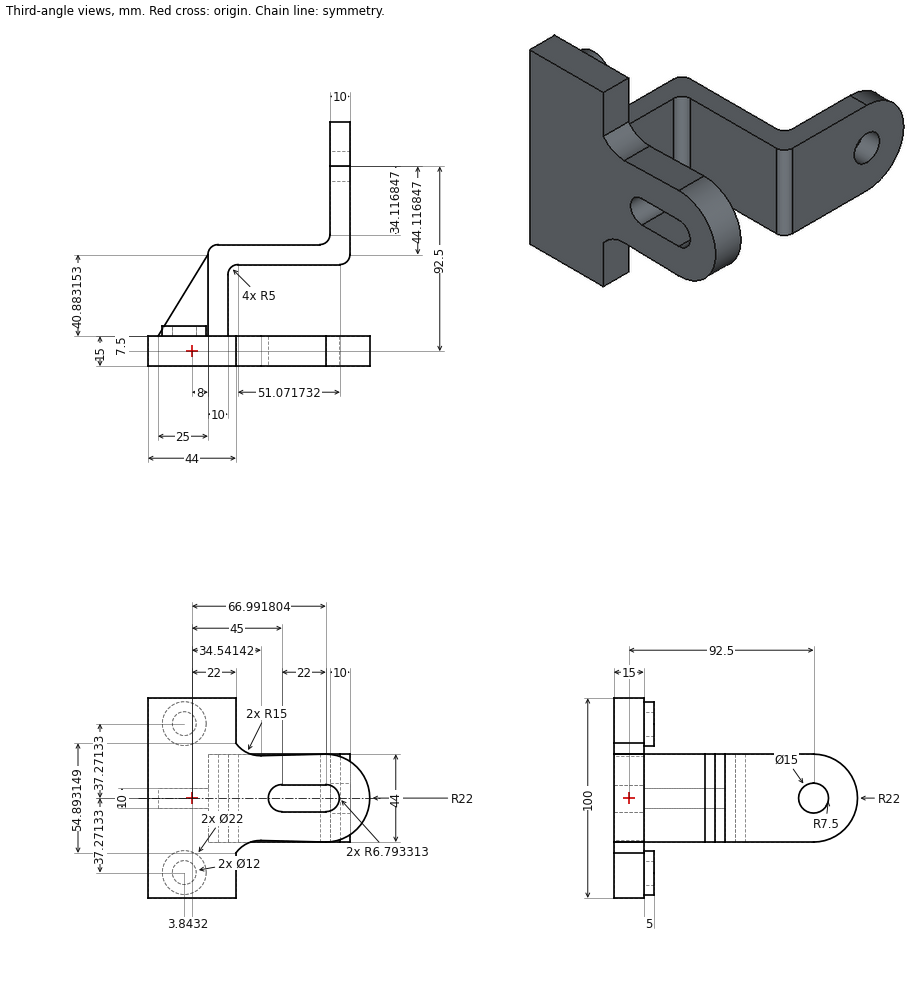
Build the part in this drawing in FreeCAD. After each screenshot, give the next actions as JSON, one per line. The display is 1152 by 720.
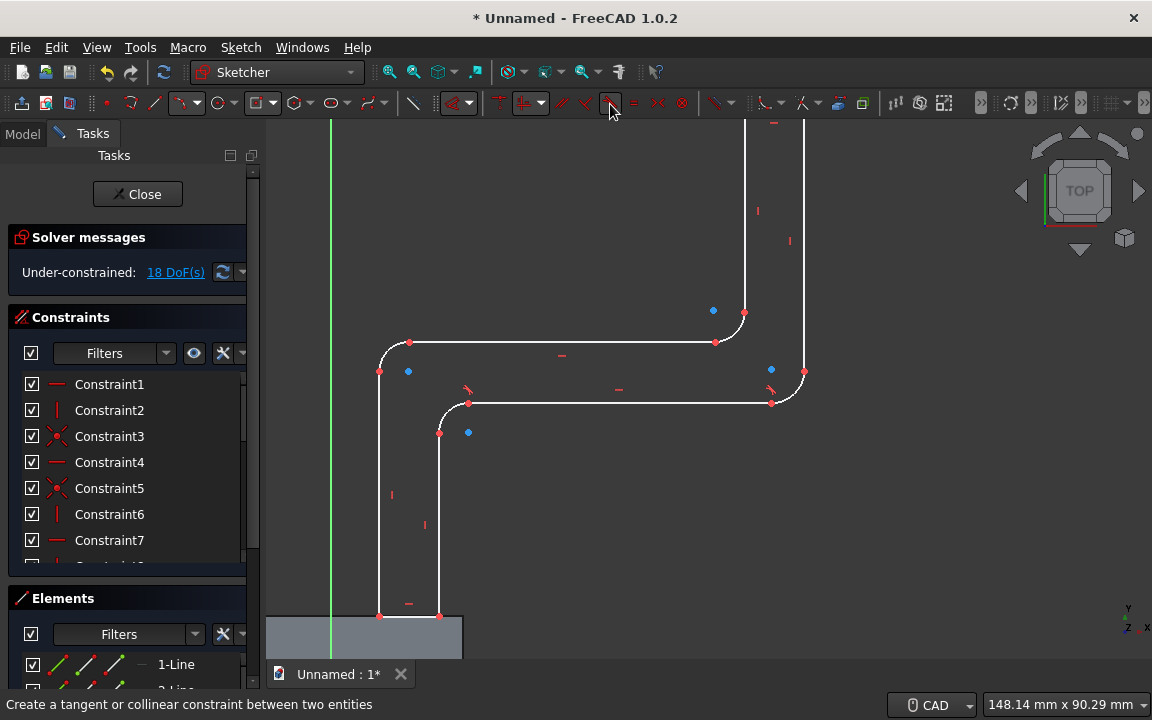
{"action": "left_click", "coordinate": [804, 293]}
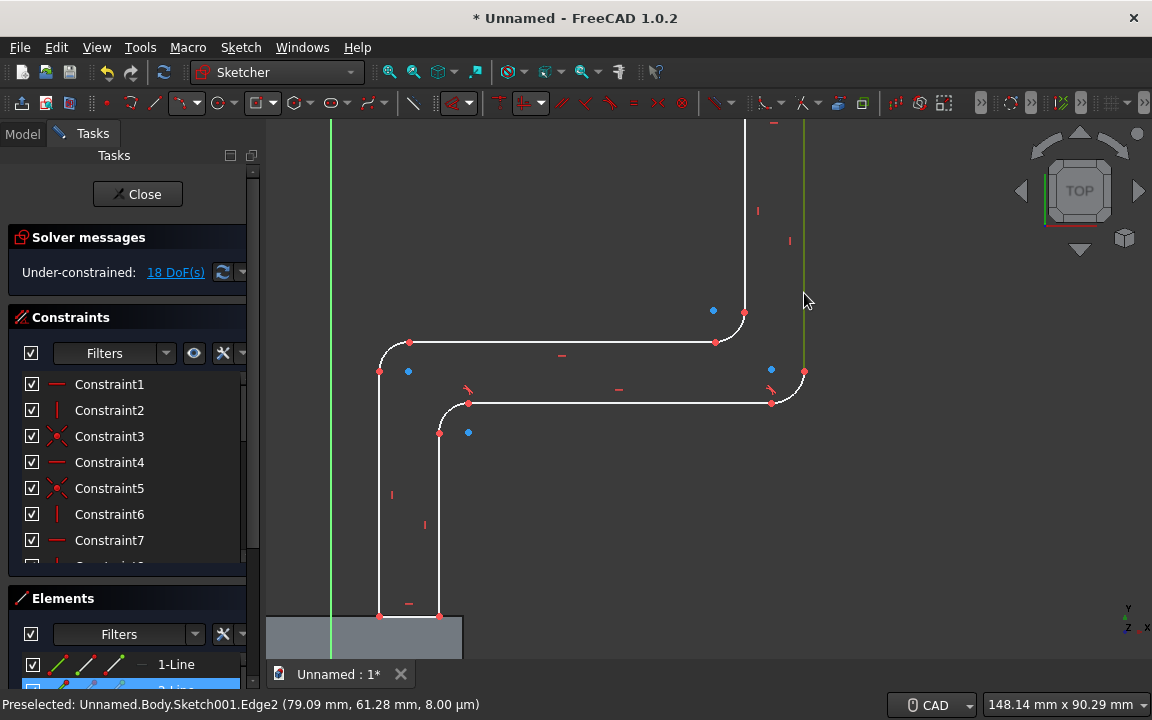
{"action": "left_click", "coordinate": [786, 400]}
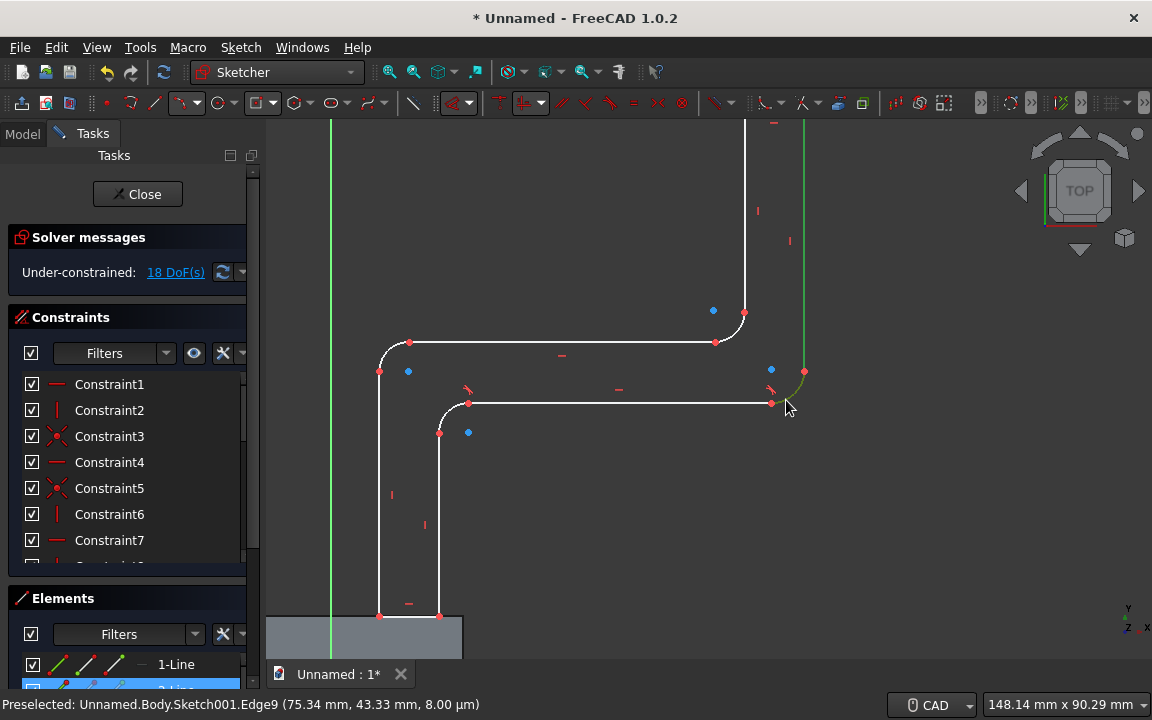
{"action": "left_click", "coordinate": [610, 104]}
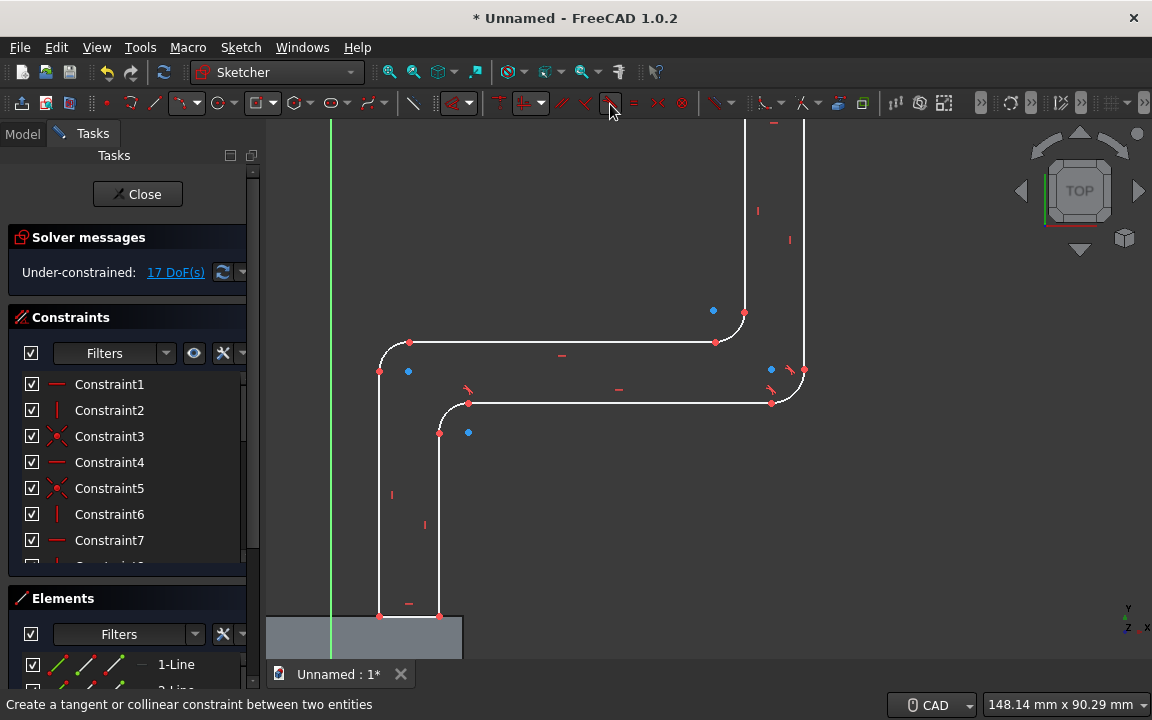
{"action": "left_click", "coordinate": [745, 170]}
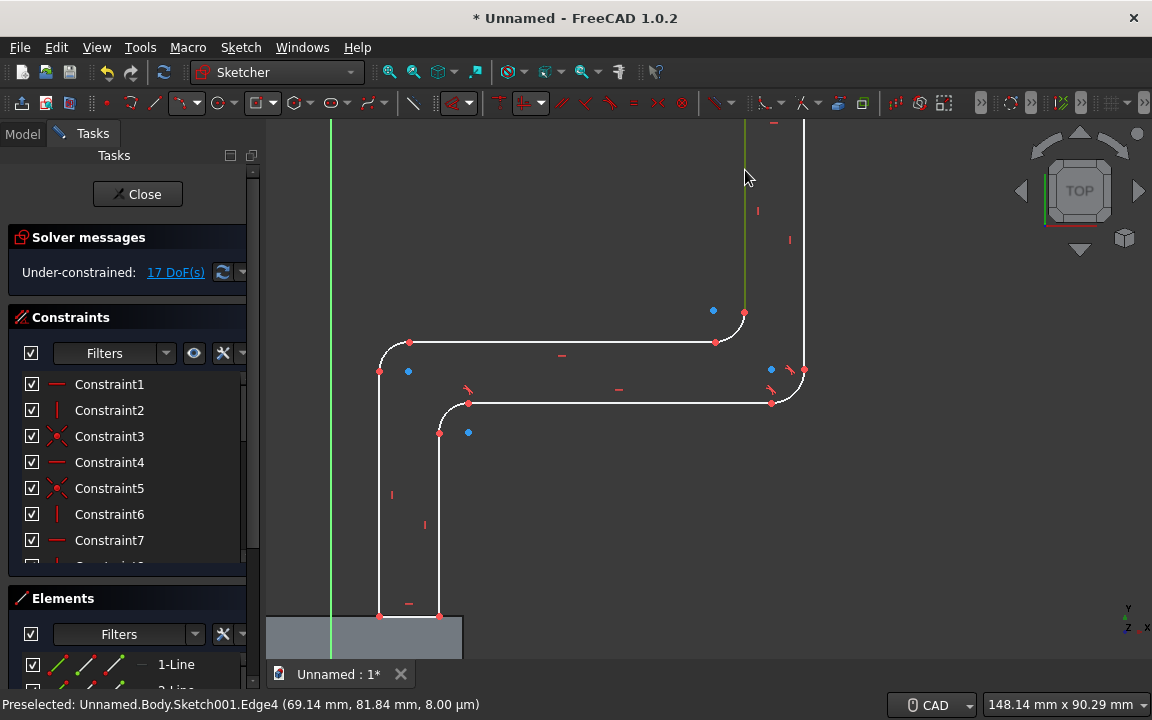
{"action": "left_click", "coordinate": [728, 338]}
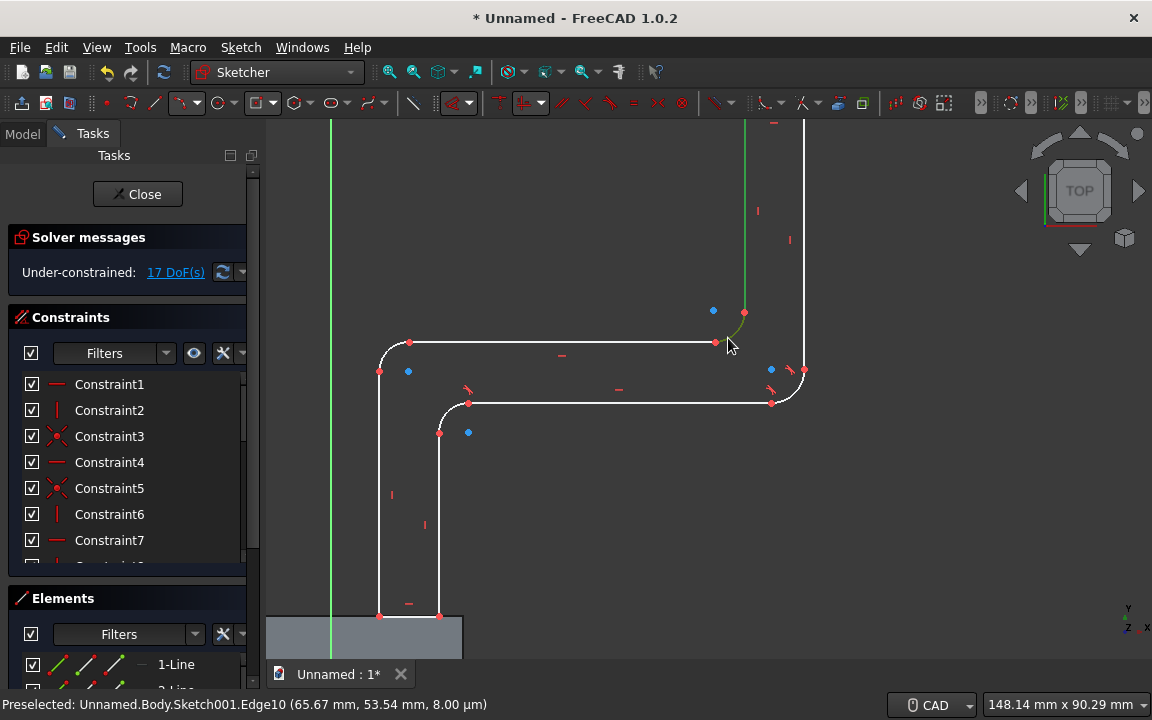
{"action": "left_click", "coordinate": [610, 104]}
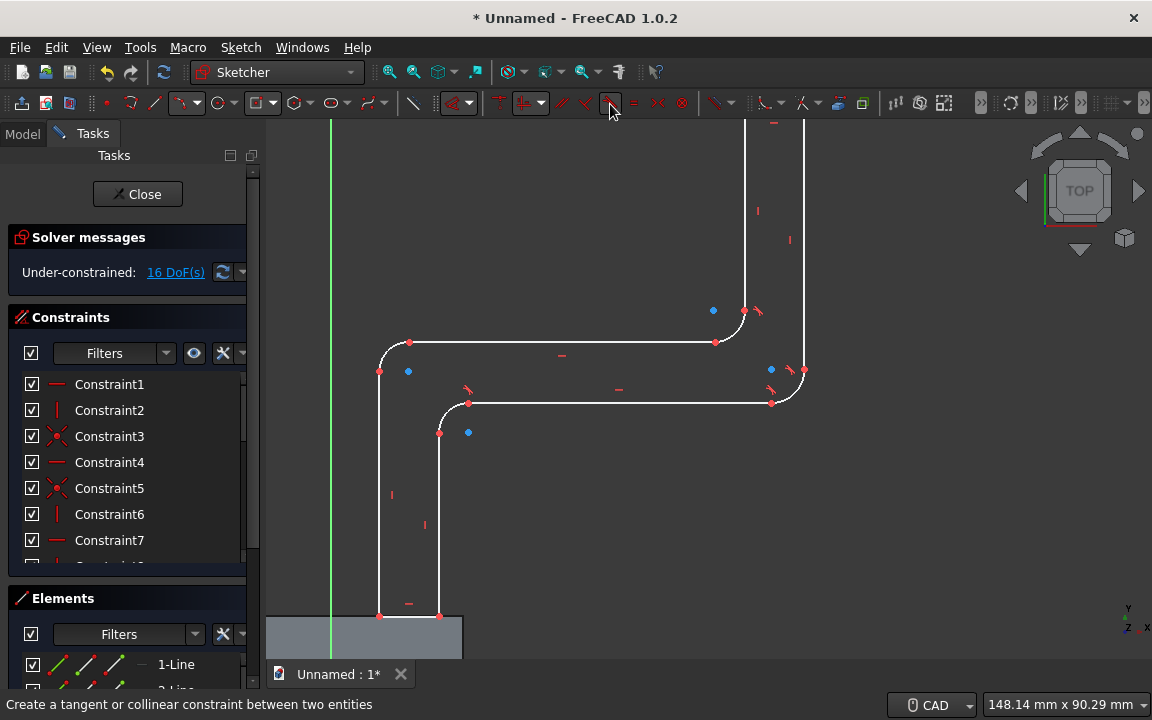
{"action": "left_click", "coordinate": [623, 342]}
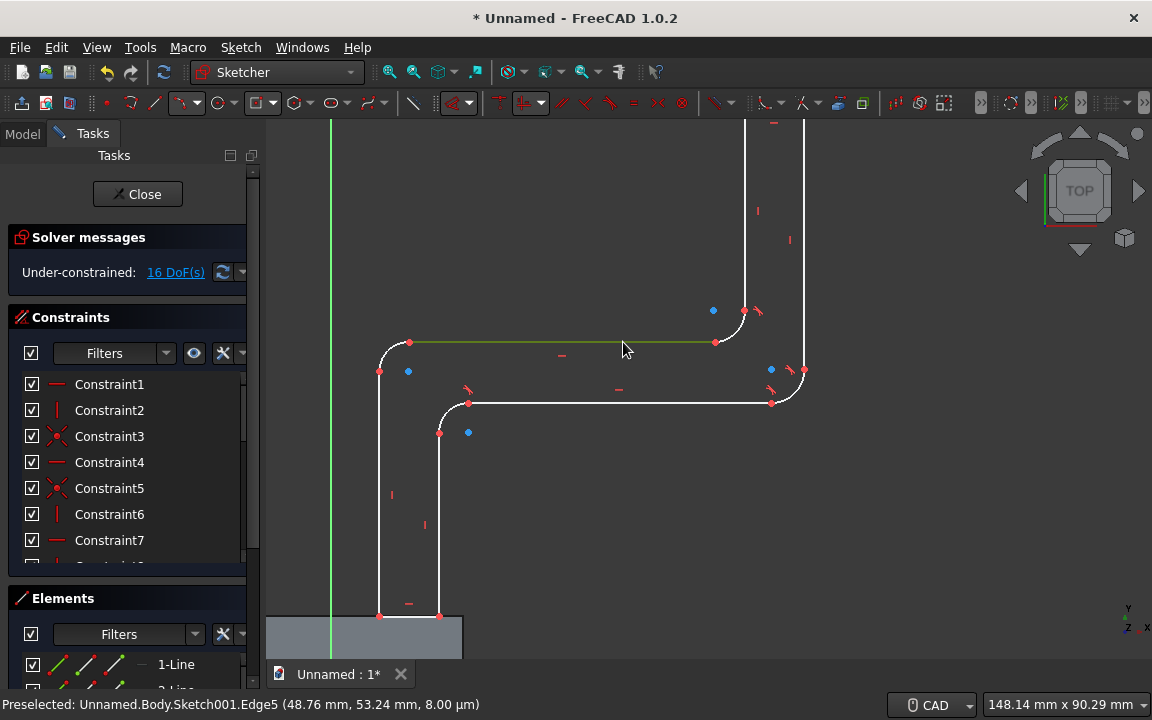
{"action": "left_click", "coordinate": [729, 338]}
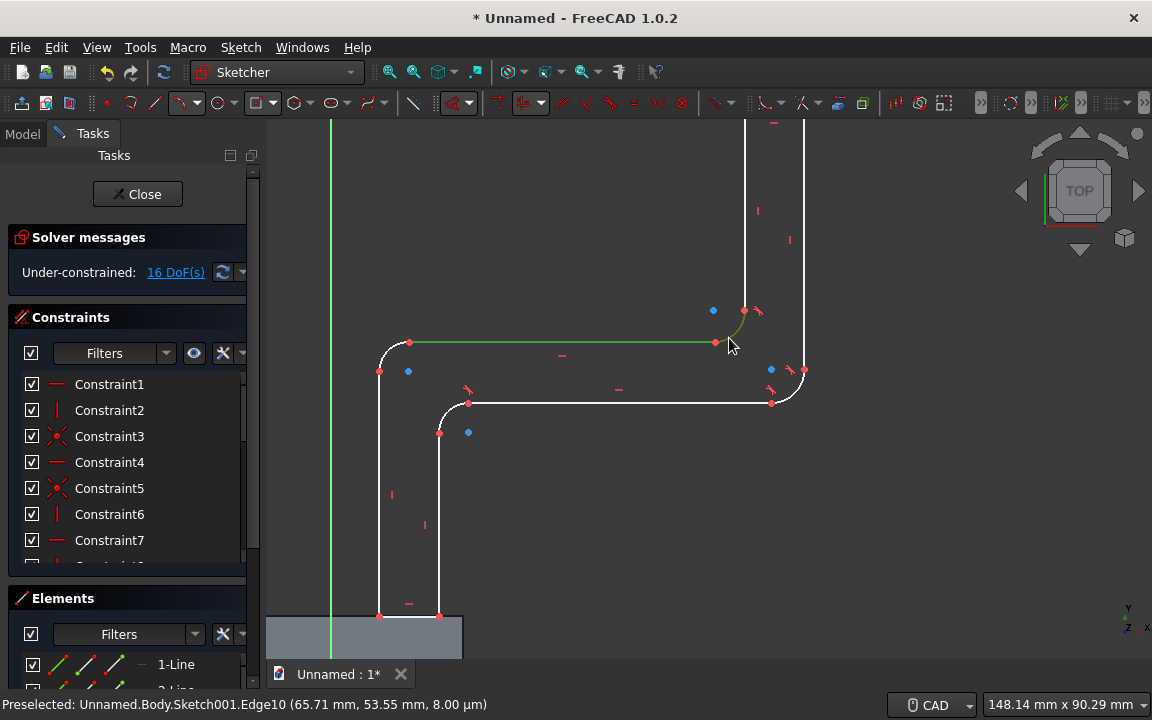
{"action": "left_click", "coordinate": [610, 104]}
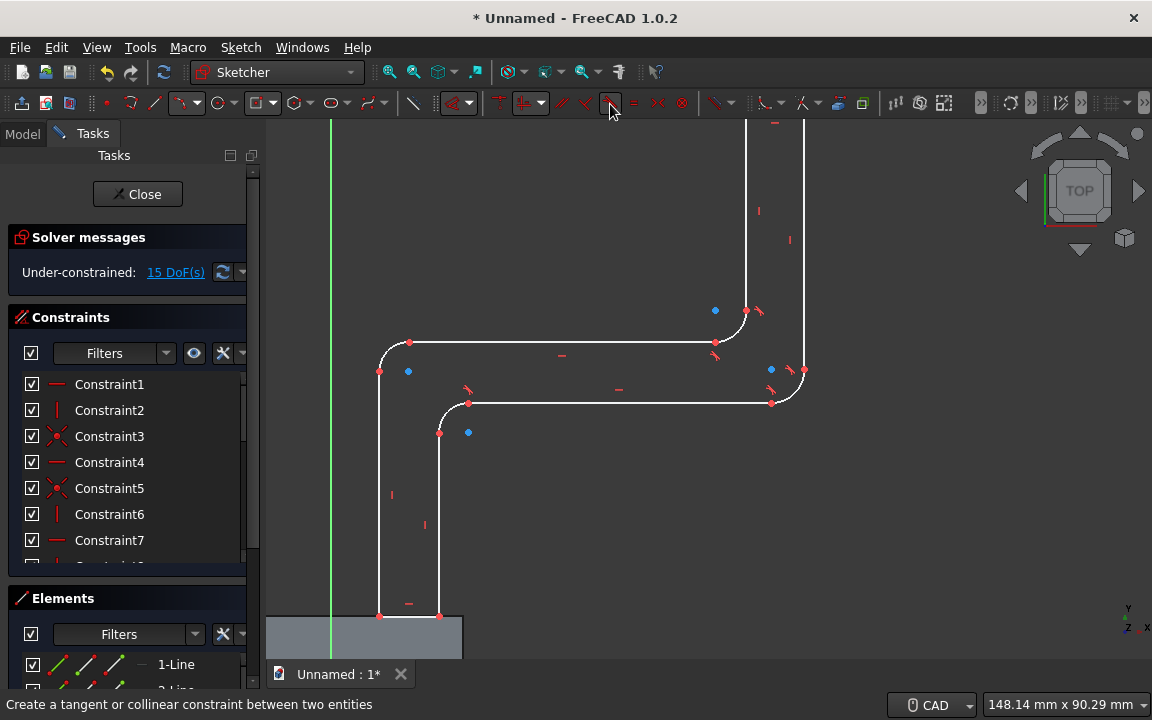
{"action": "left_click", "coordinate": [623, 342]}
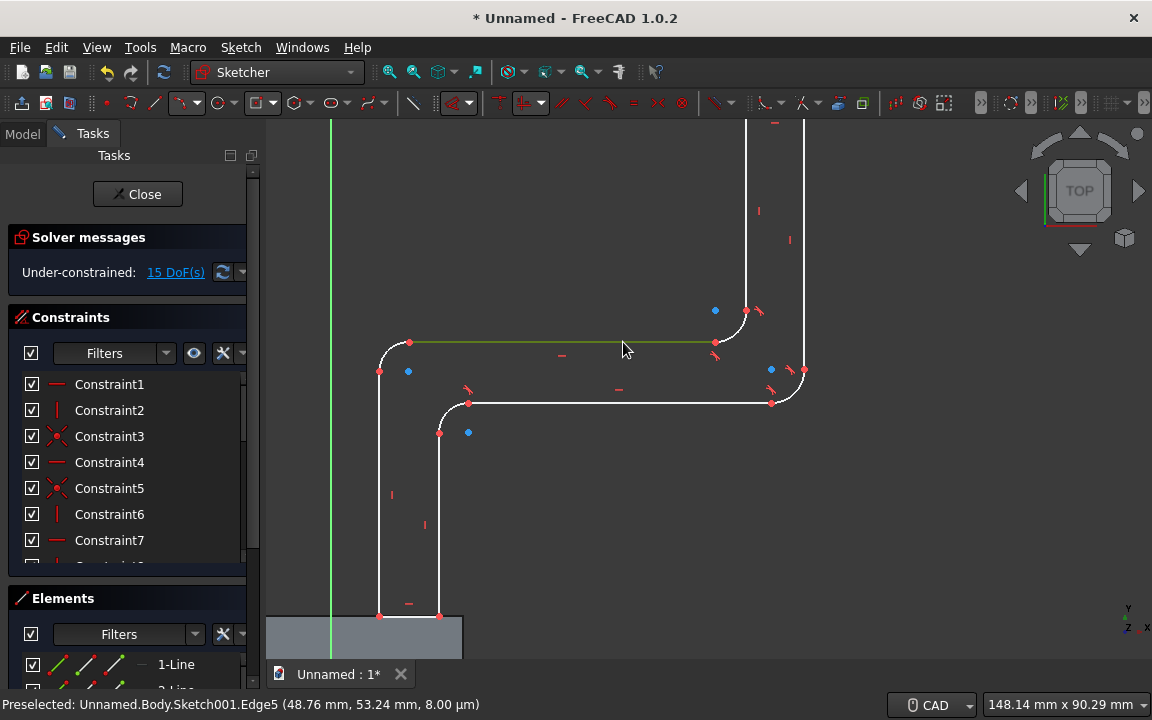
{"action": "left_click", "coordinate": [396, 345]}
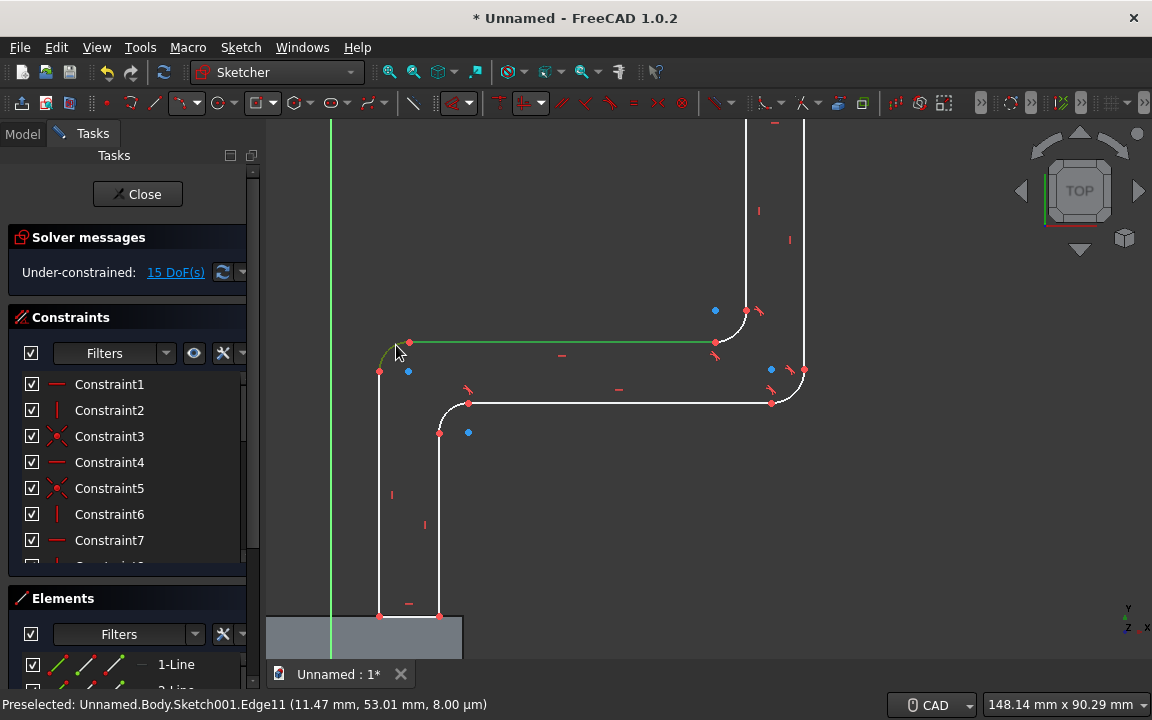
{"action": "left_click", "coordinate": [610, 104]}